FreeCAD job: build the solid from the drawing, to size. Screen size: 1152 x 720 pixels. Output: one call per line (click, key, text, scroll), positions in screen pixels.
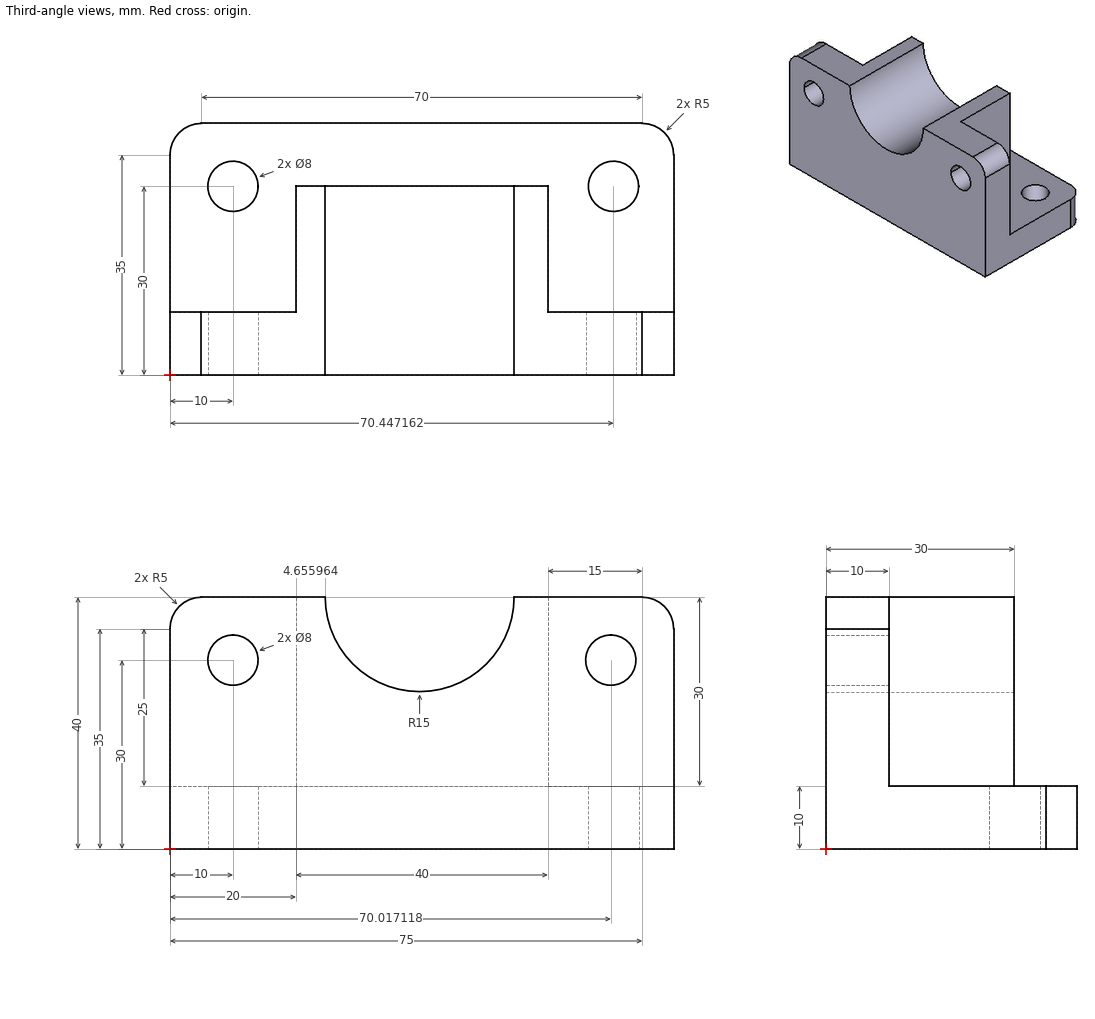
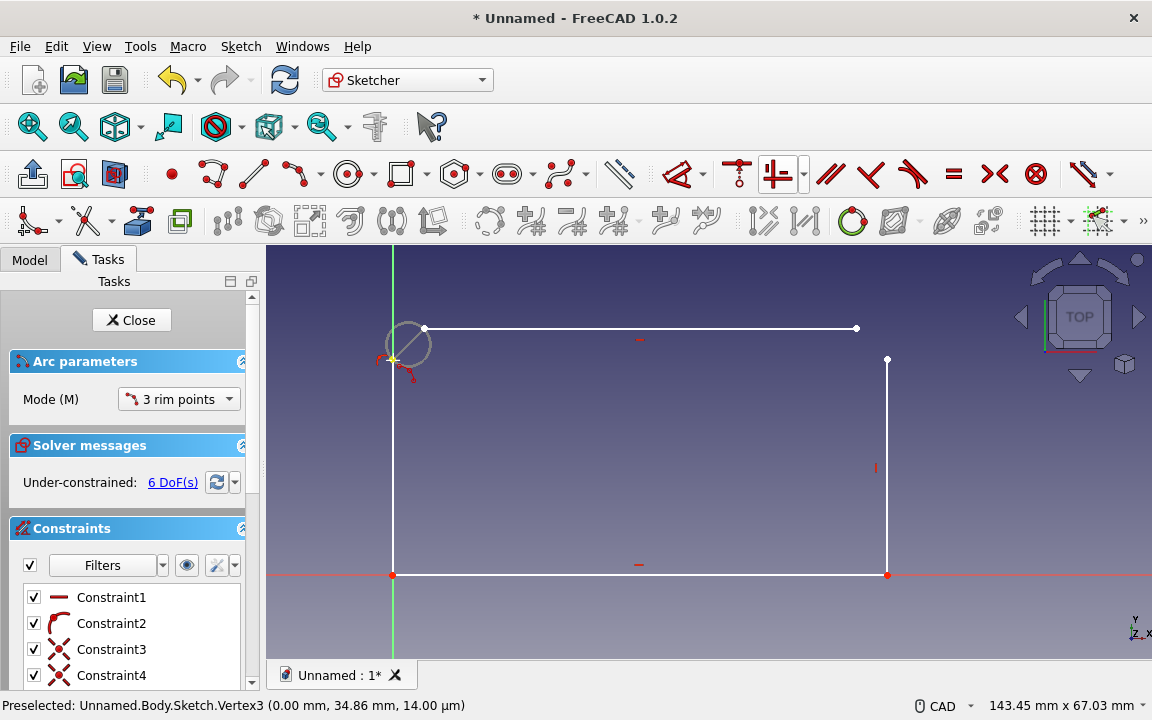
scroll(402, 337, up, 3)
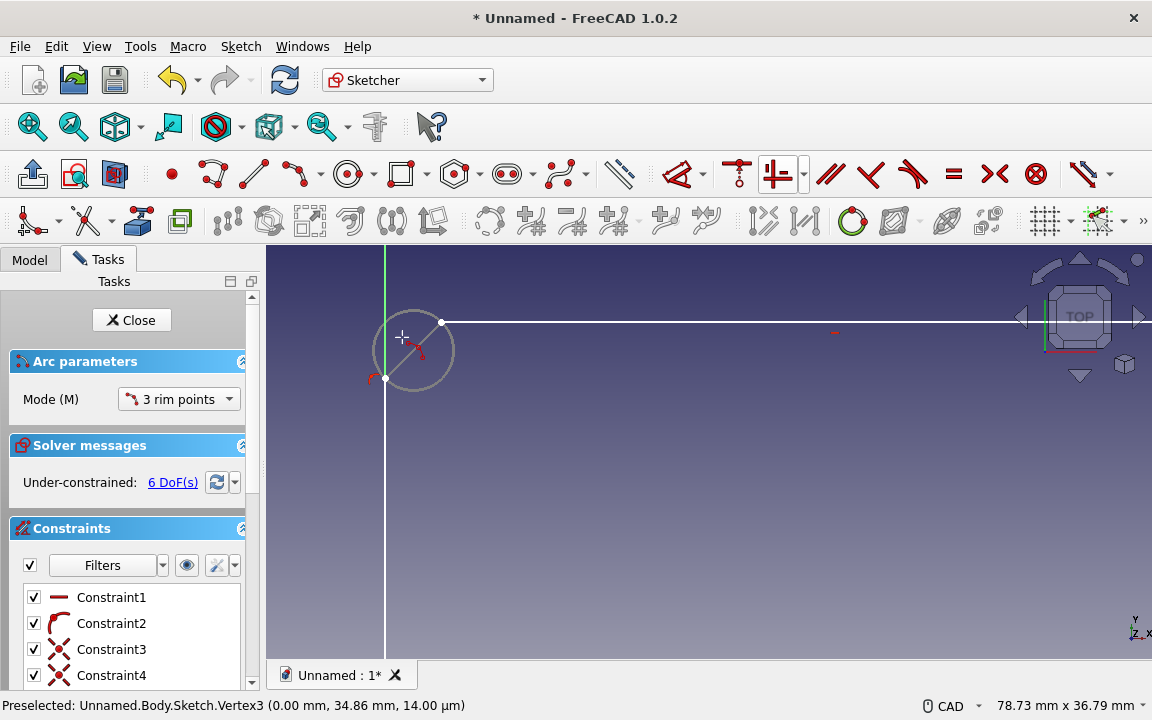
click(402, 337)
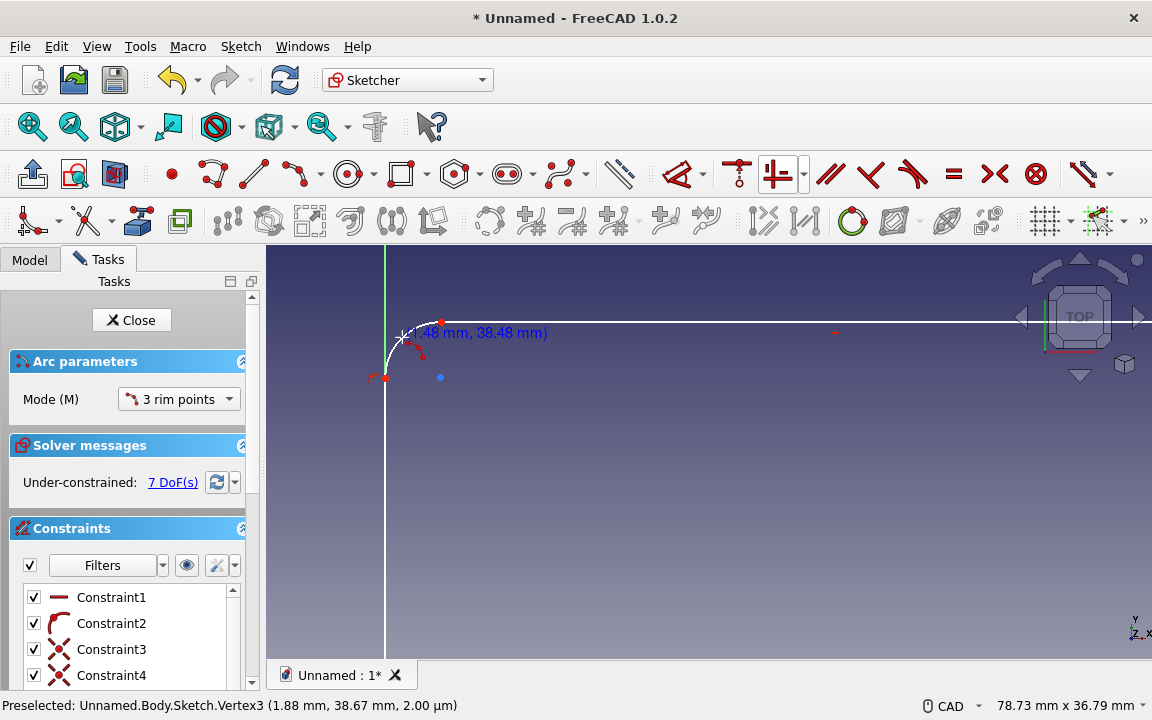
scroll(403, 338, down, 3)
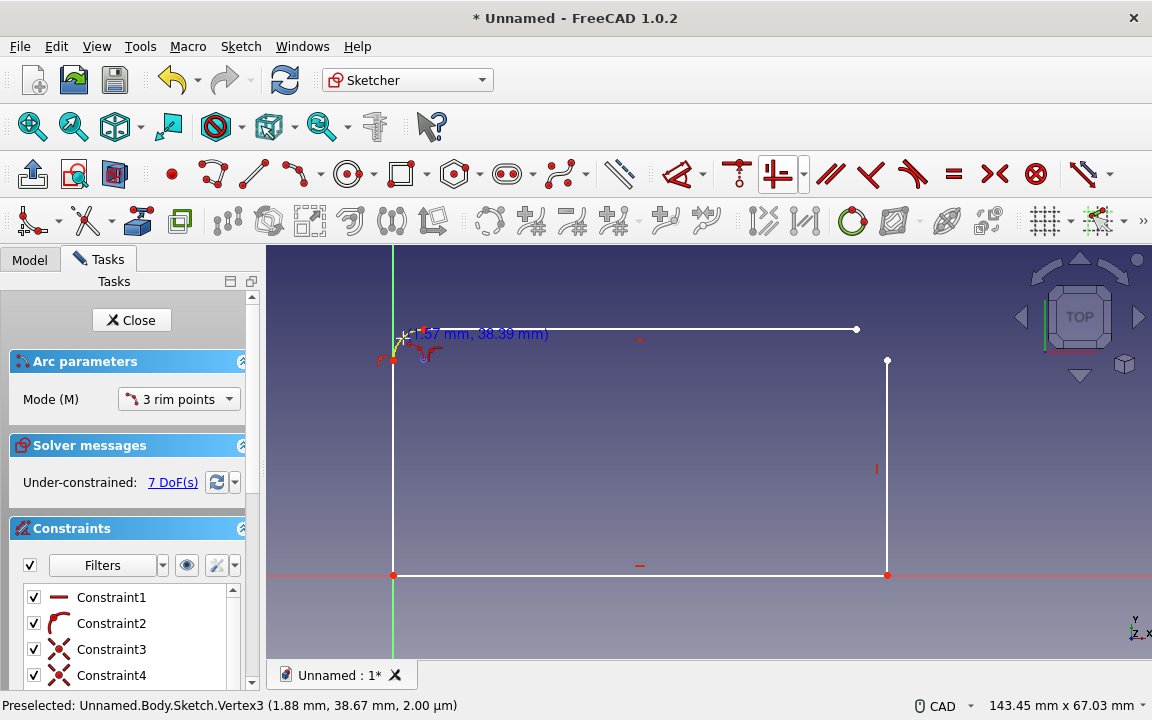
click(887, 360)
click(856, 329)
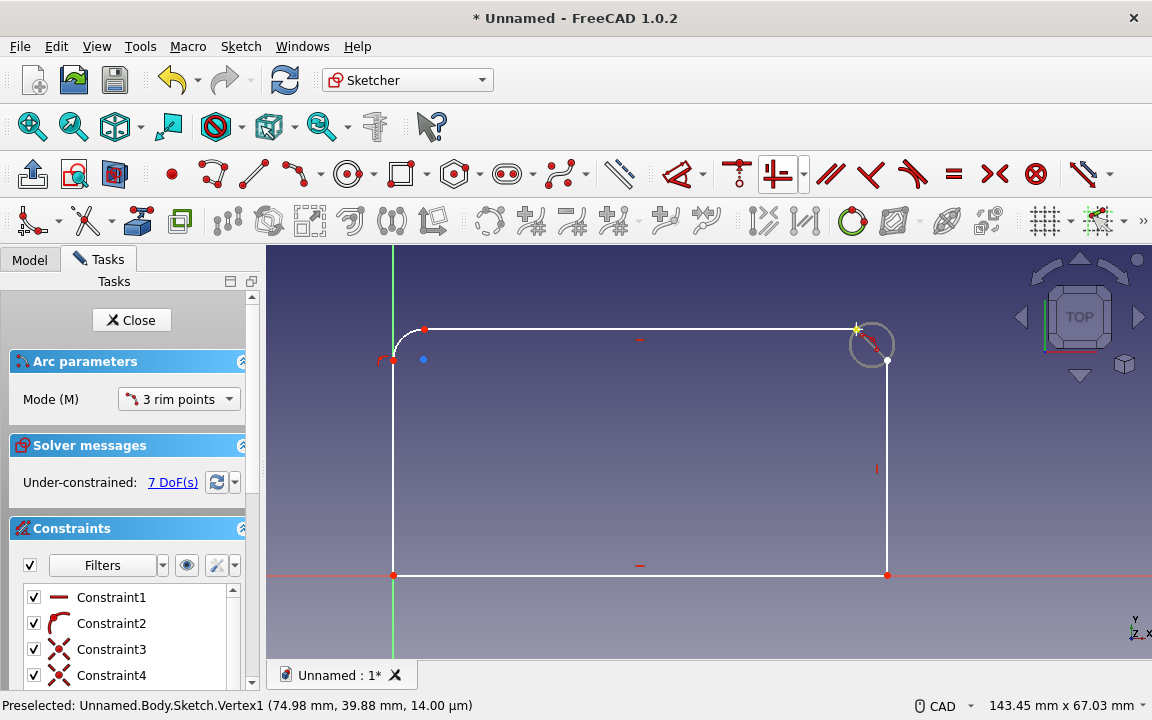
scroll(878, 338, up, 3)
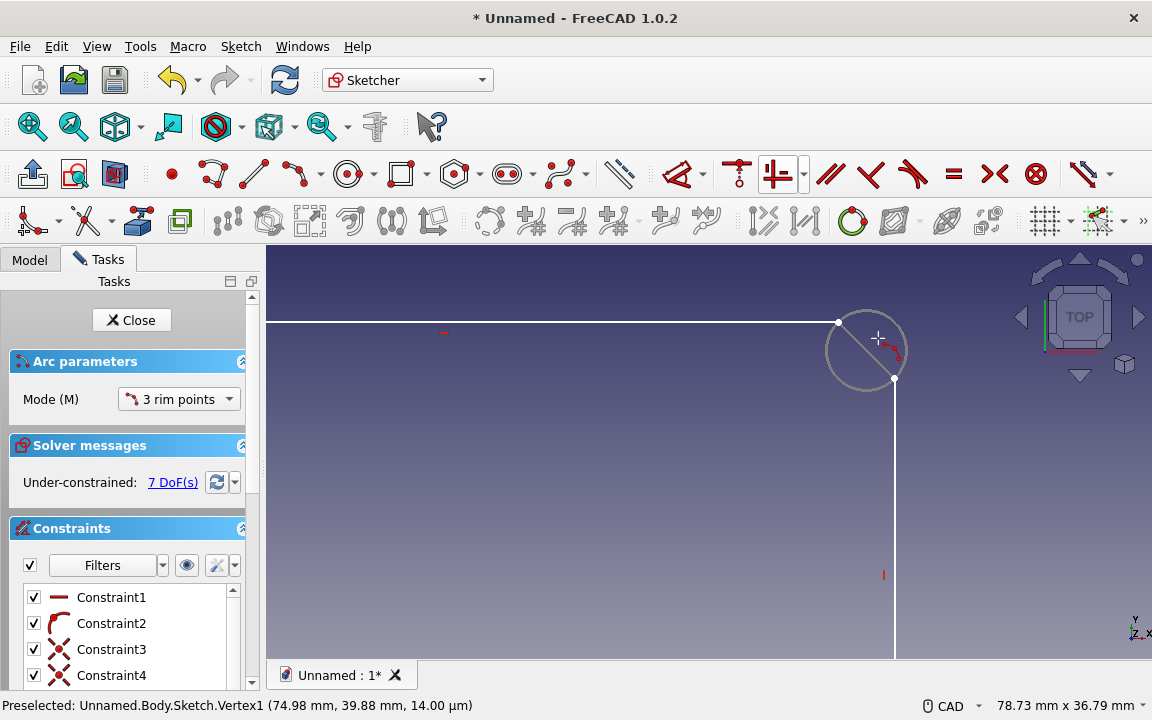
click(878, 337)
key(Escape)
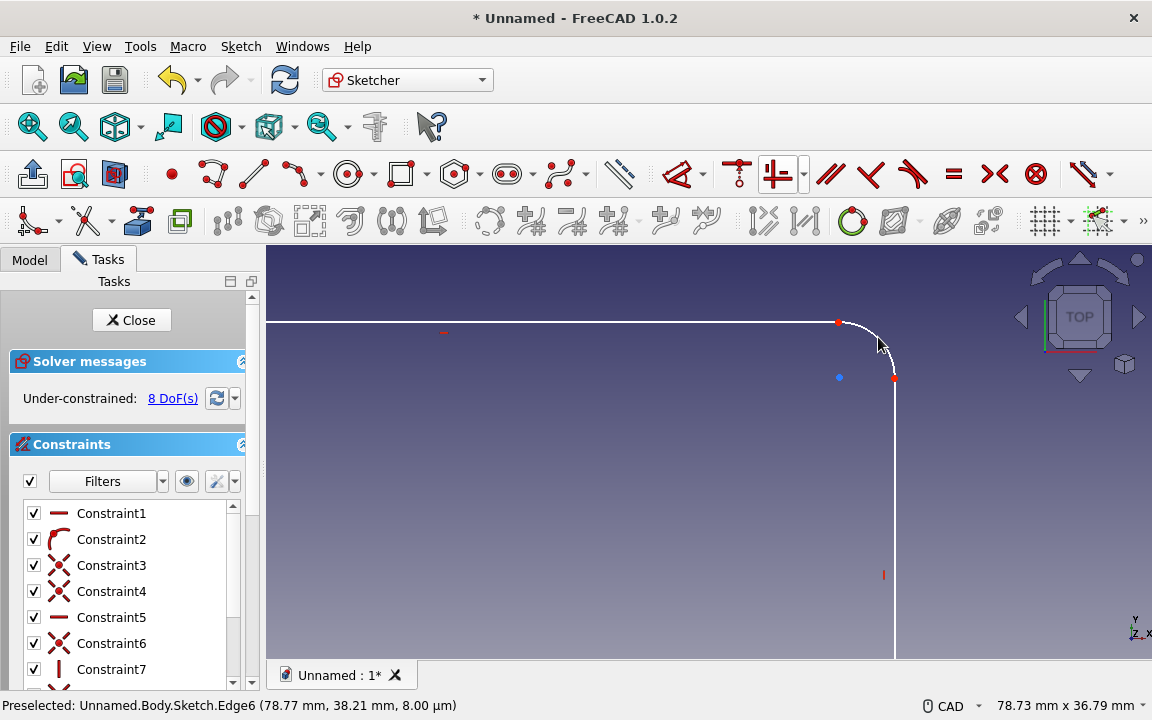
click(602, 322)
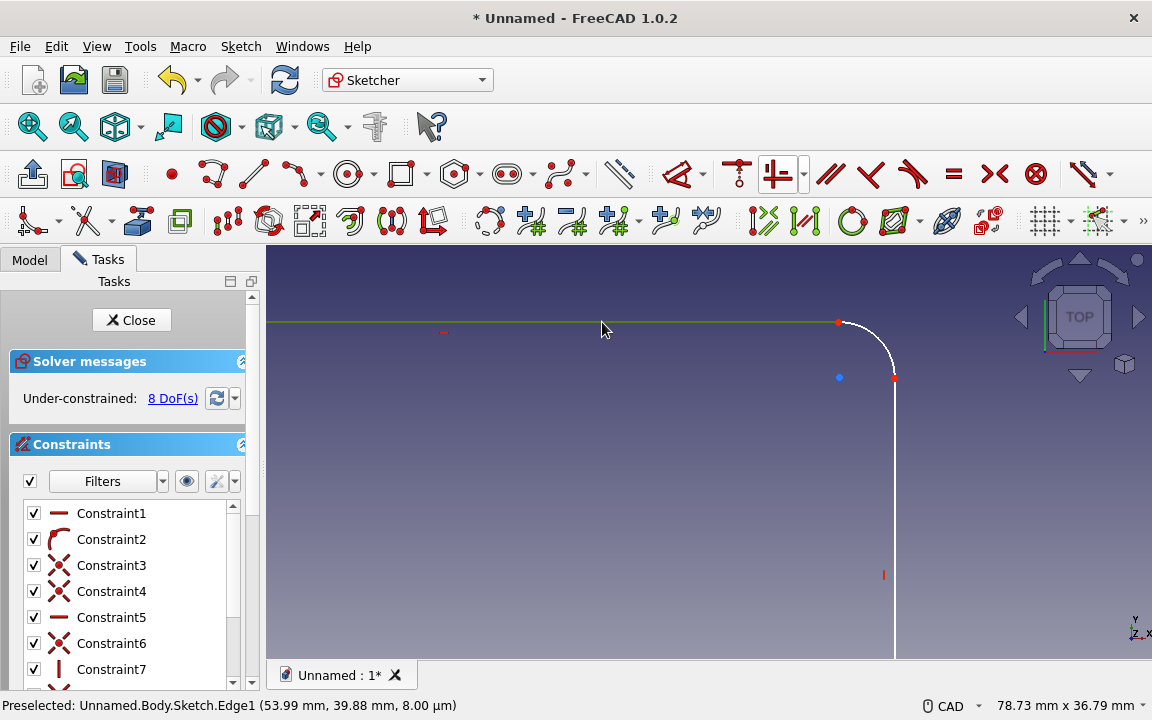
scroll(879, 338, down, 3)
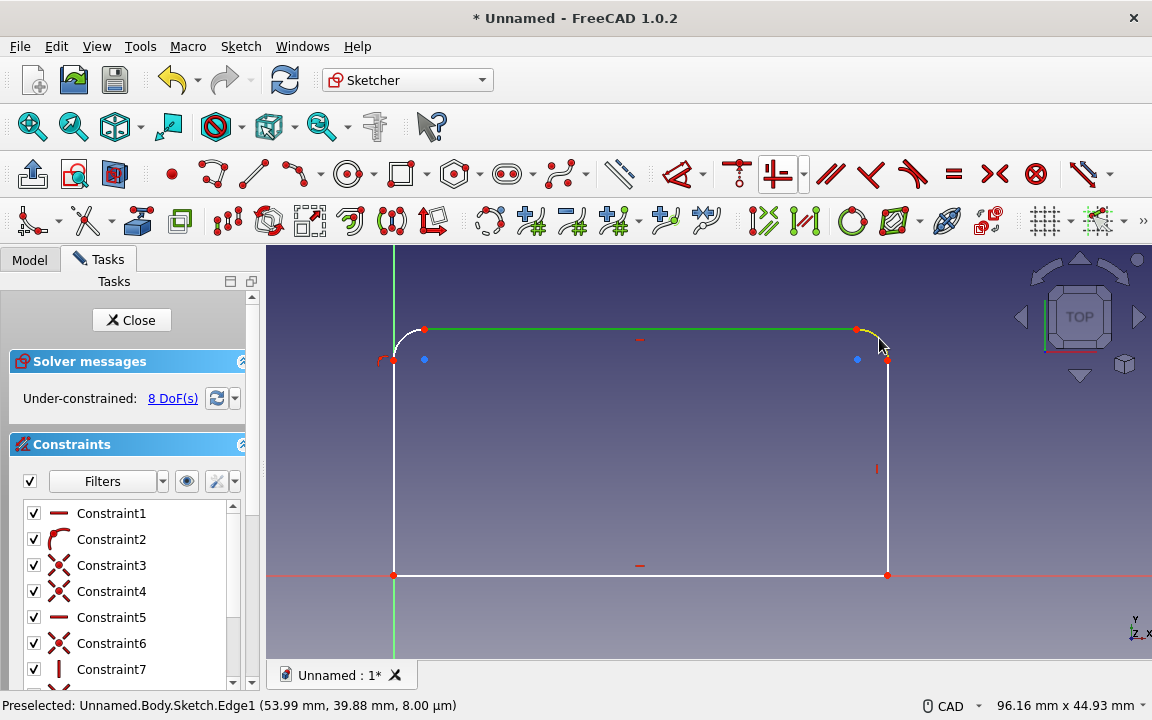
click(411, 333)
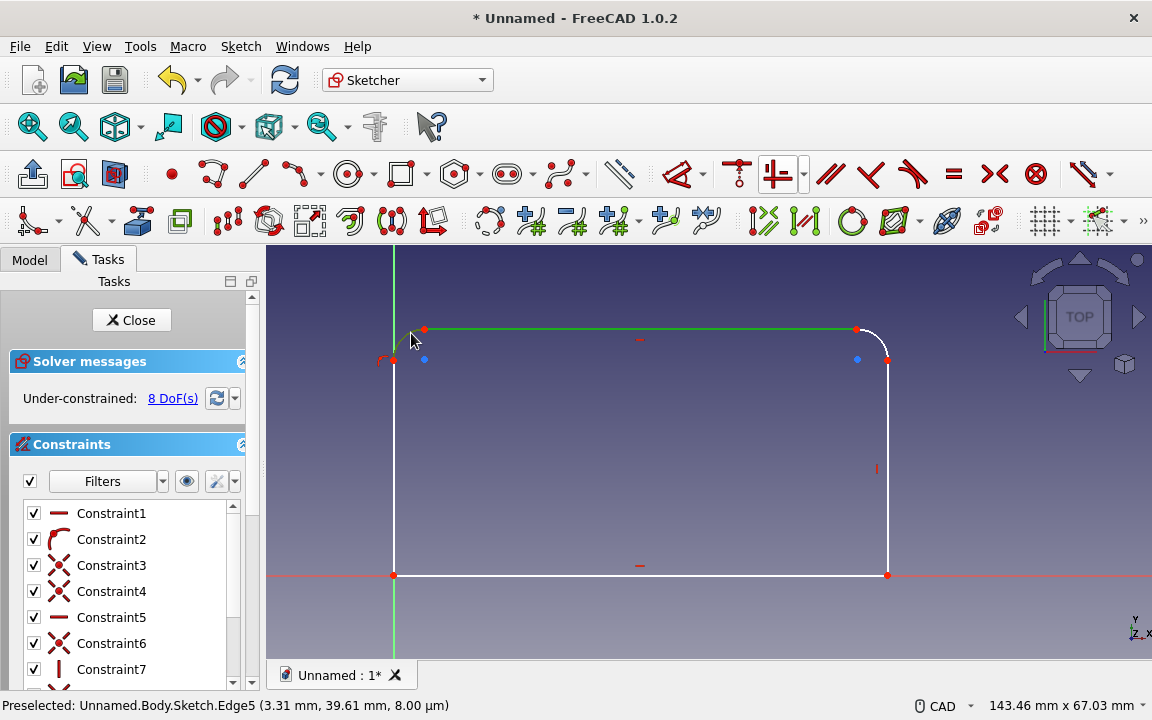
click(913, 174)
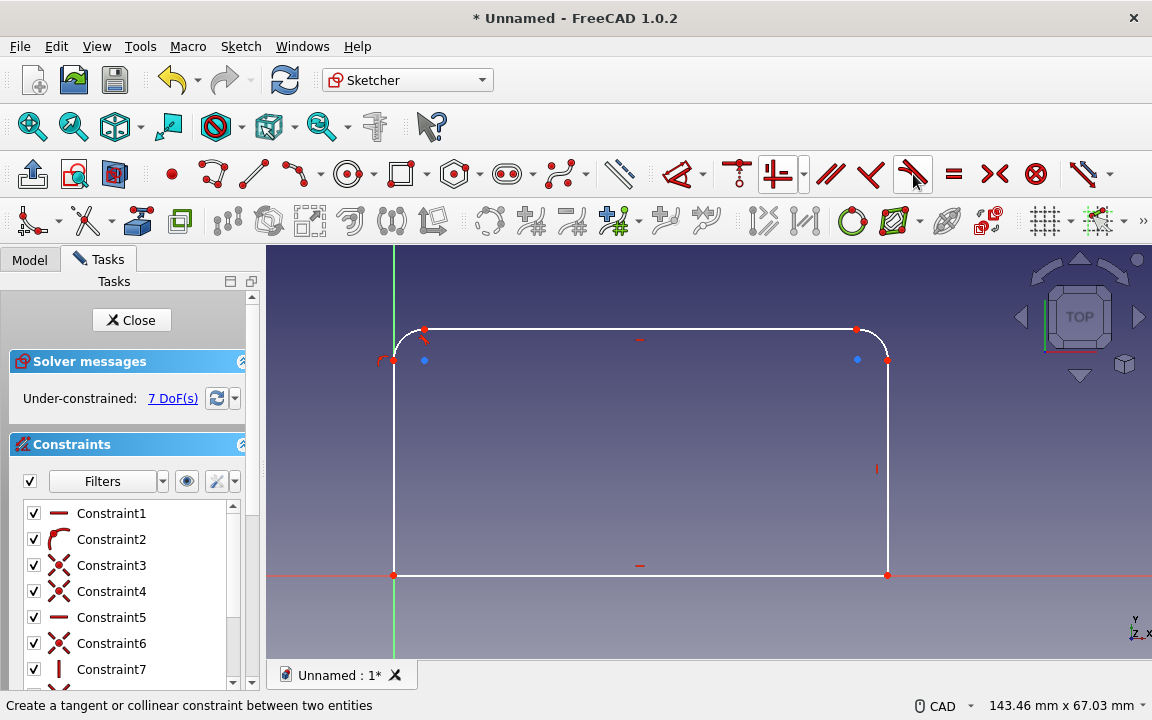
click(727, 329)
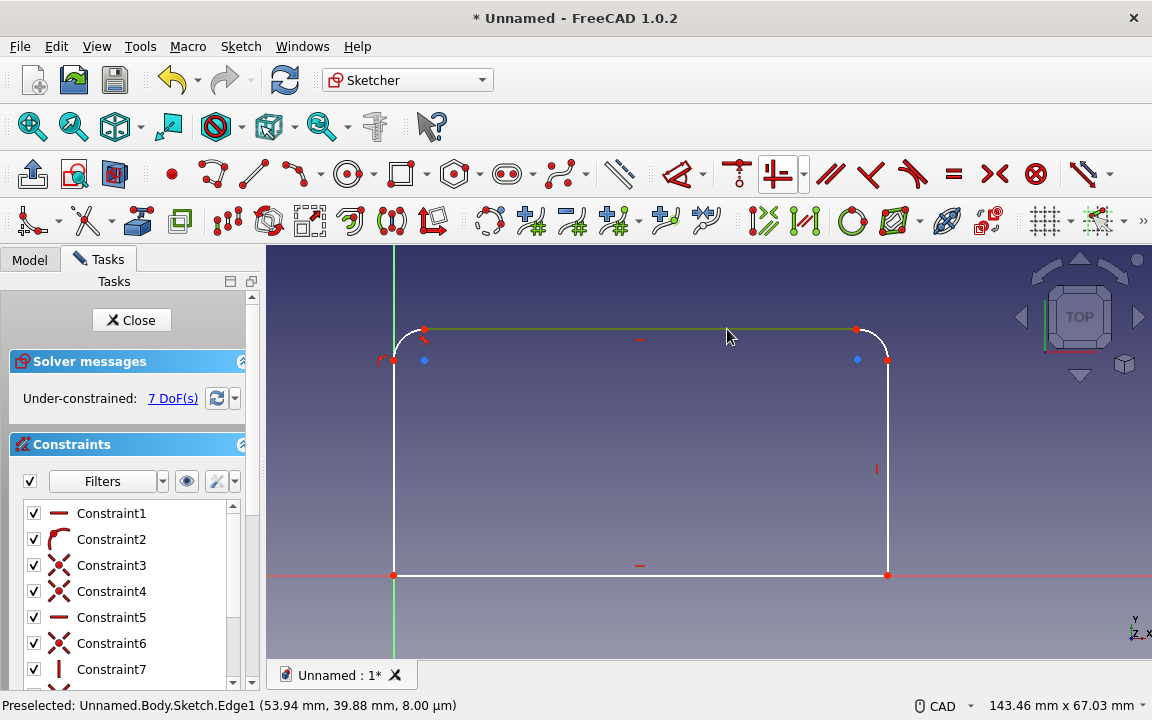
click(885, 346)